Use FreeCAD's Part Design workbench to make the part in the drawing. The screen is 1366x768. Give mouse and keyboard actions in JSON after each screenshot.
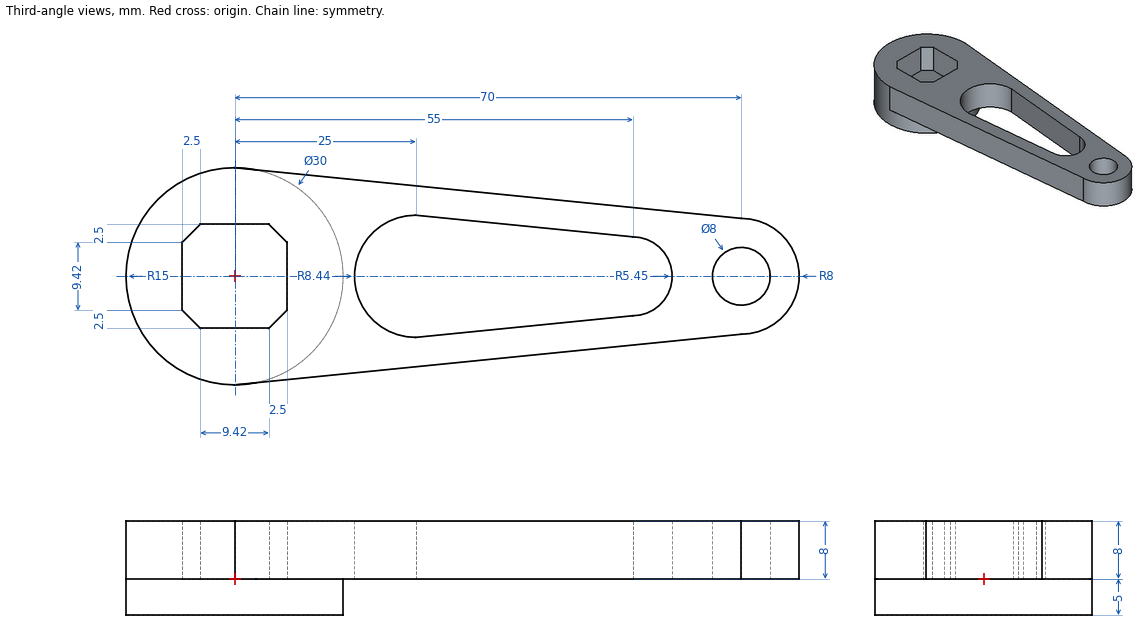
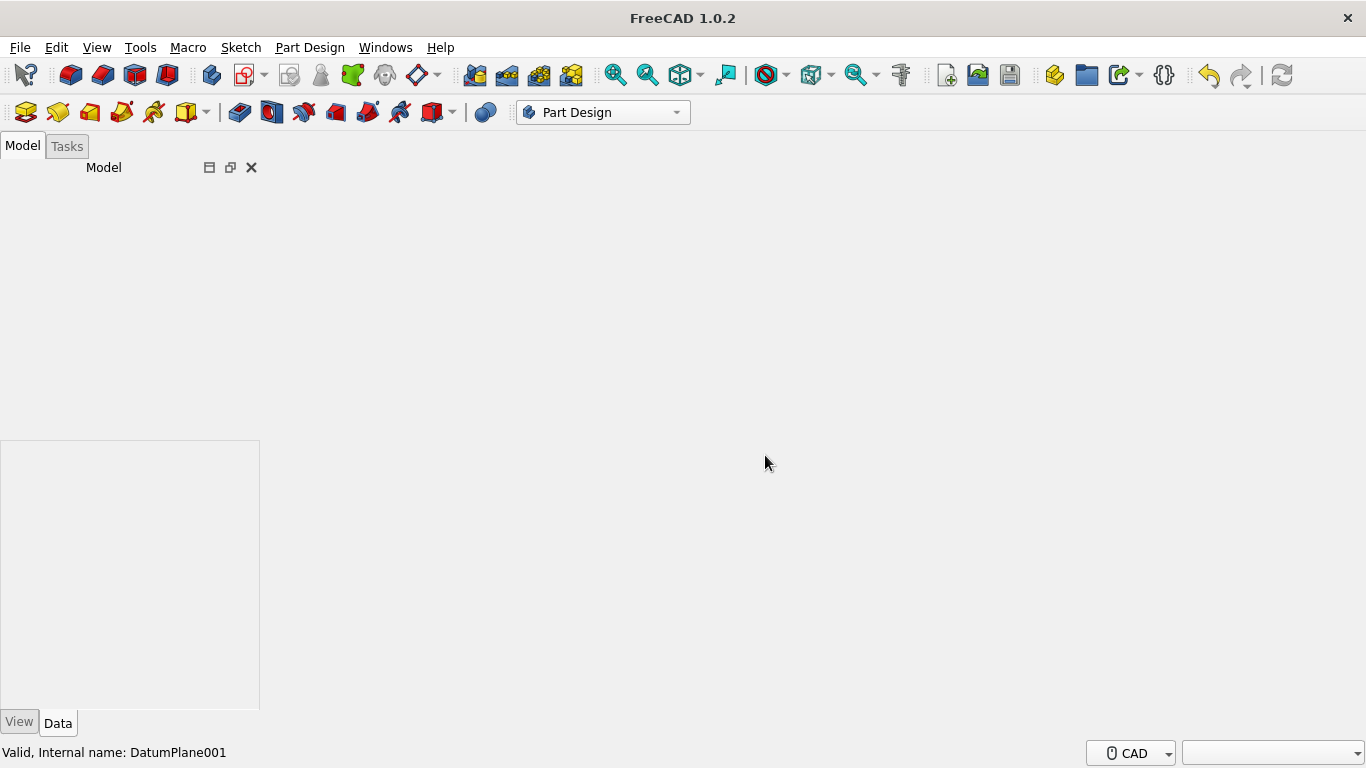
{"action": "left_click", "coordinate": [946, 76]}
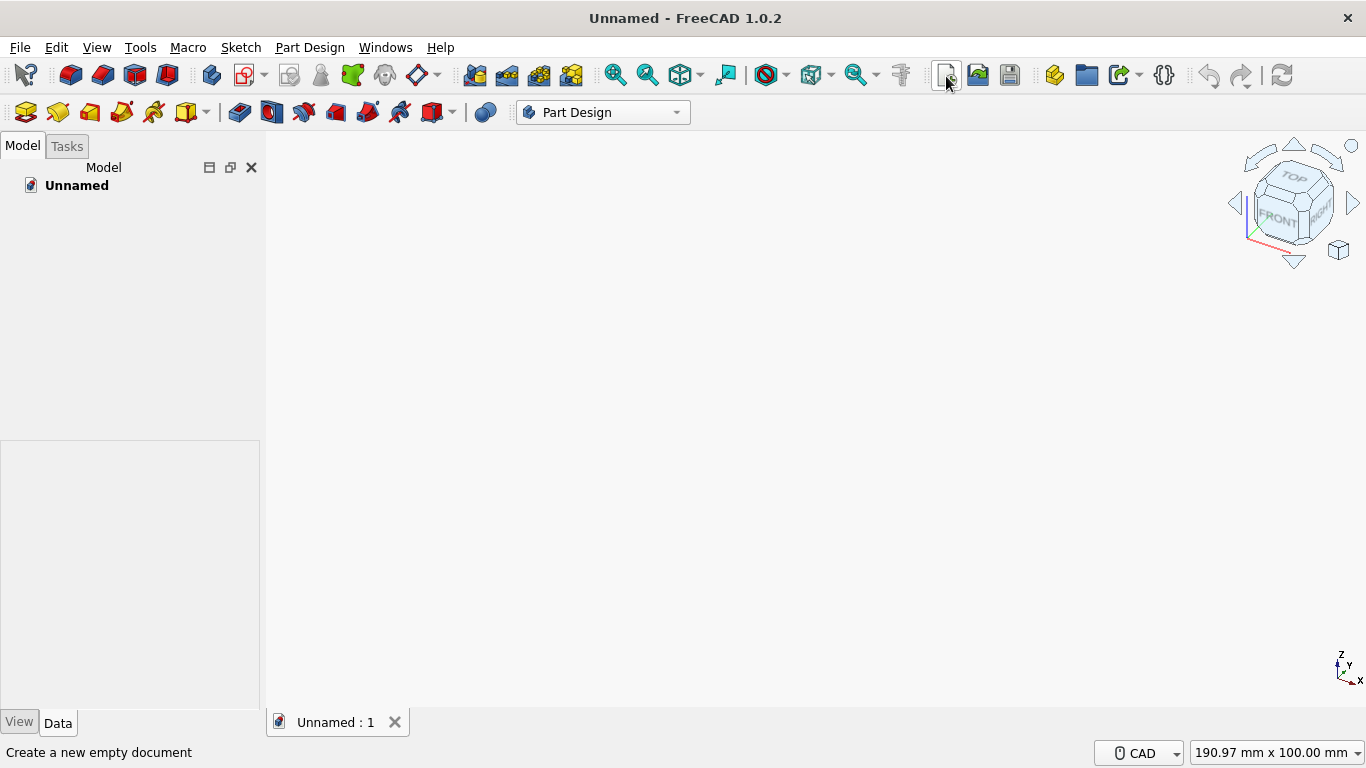
{"action": "left_click", "coordinate": [244, 76]}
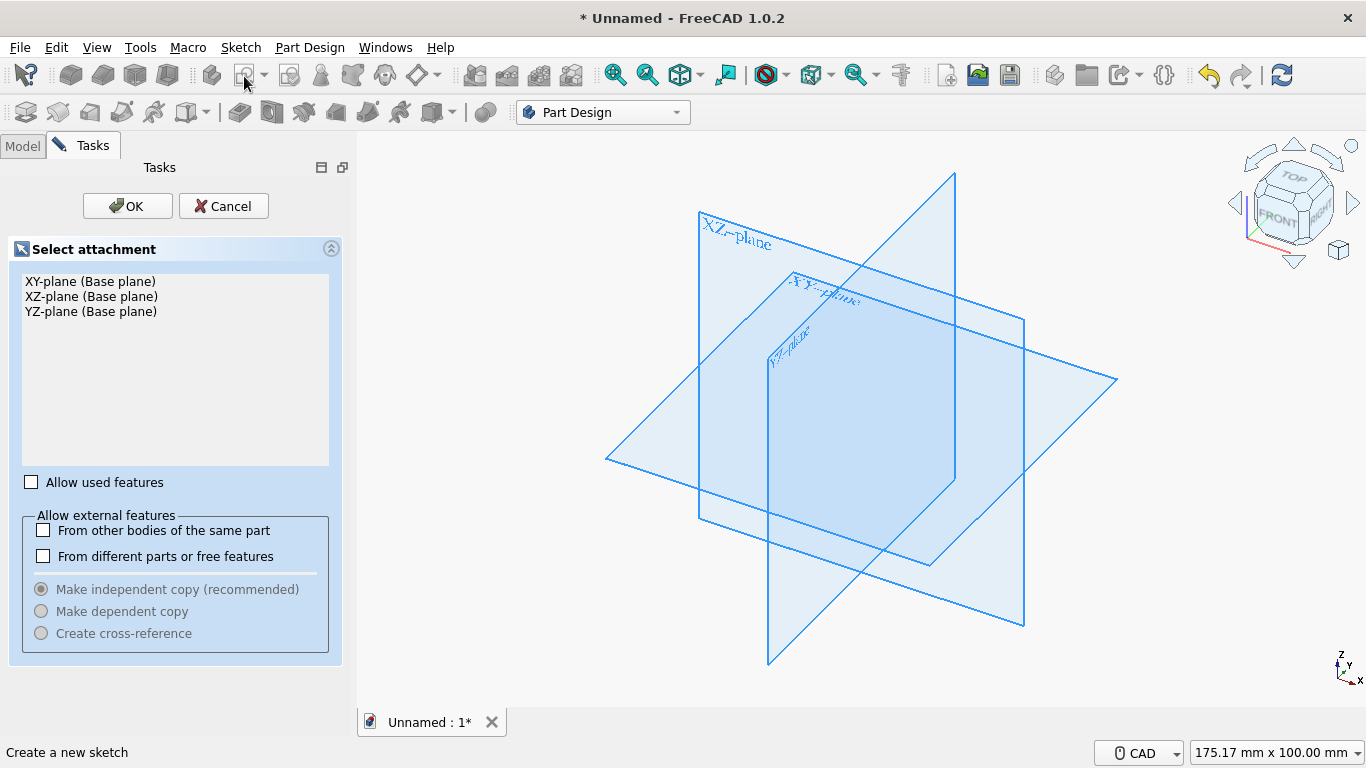
{"action": "left_click", "coordinate": [82, 282]}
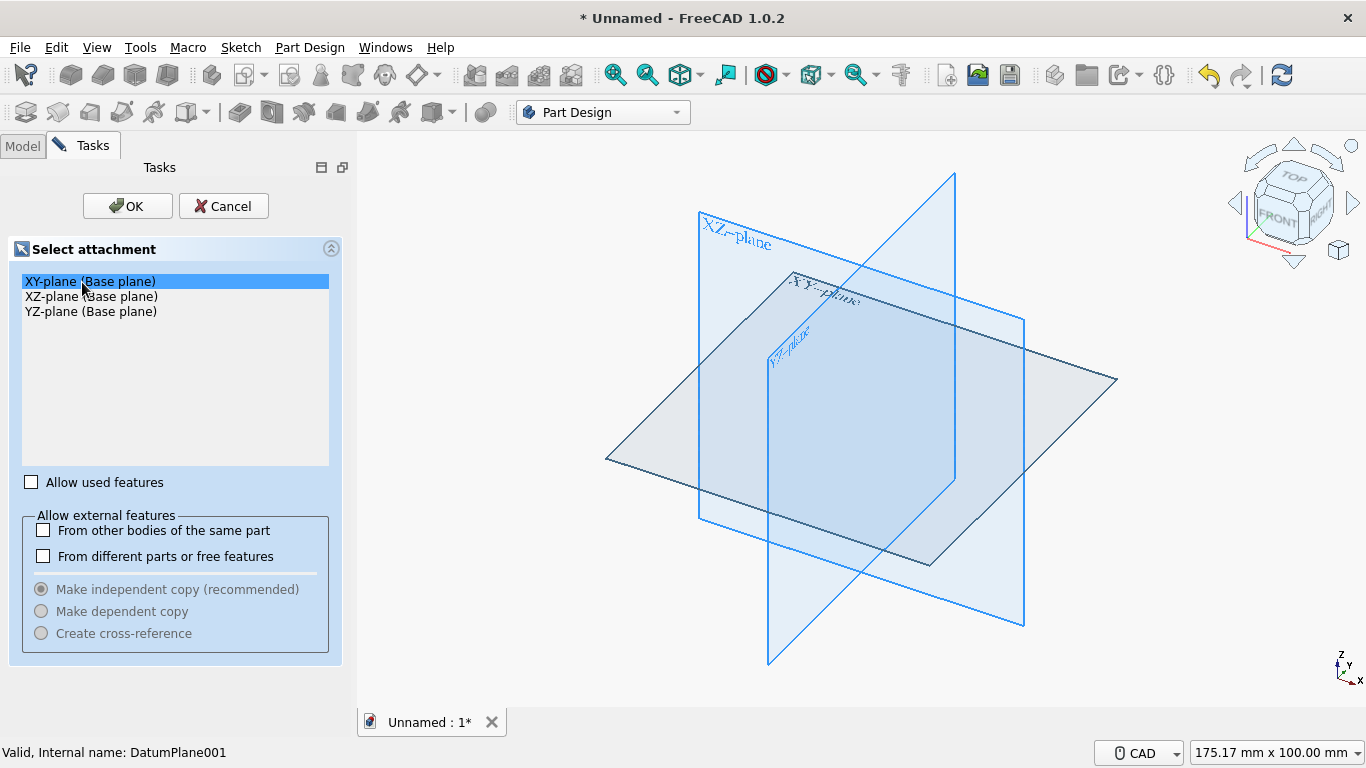
{"action": "left_click", "coordinate": [128, 206]}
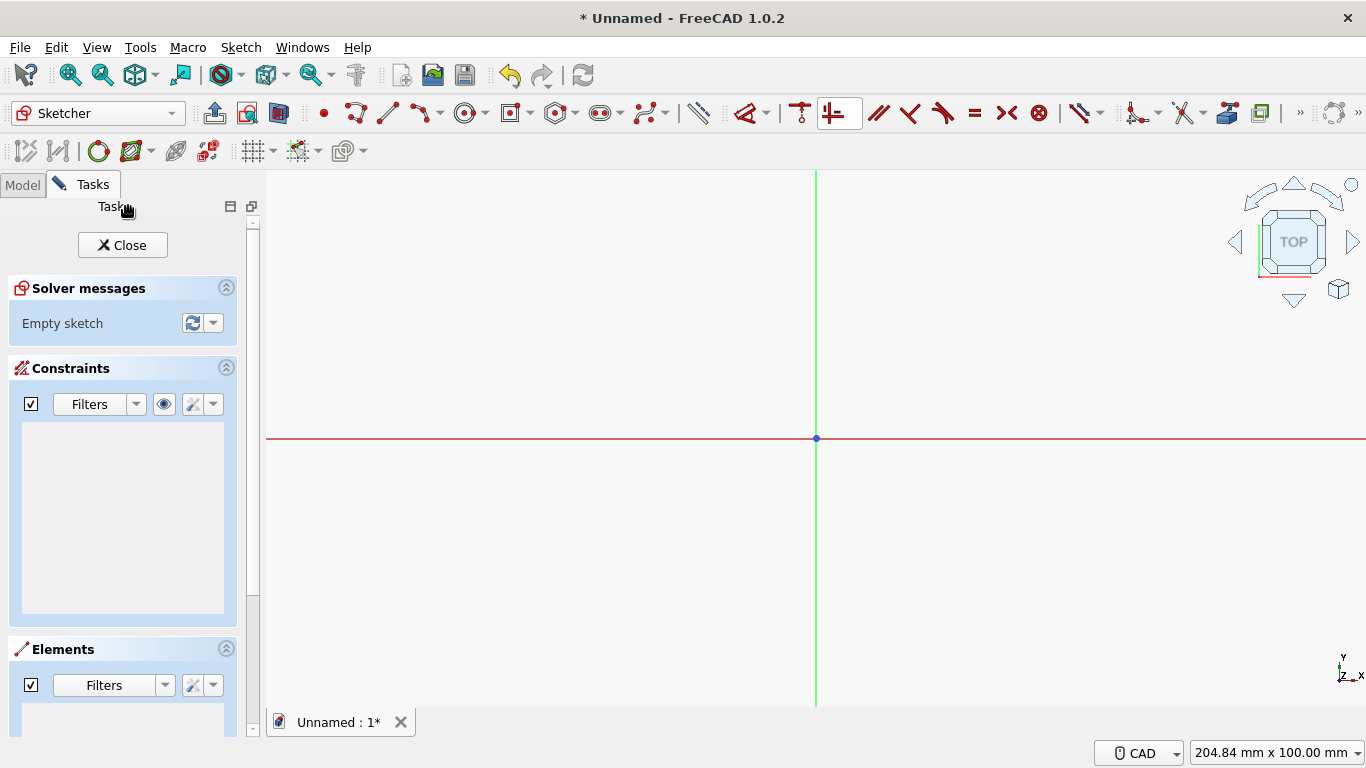
{"action": "scroll", "coordinate": [294, 439], "scroll_direction": "down", "scroll_amount": 1}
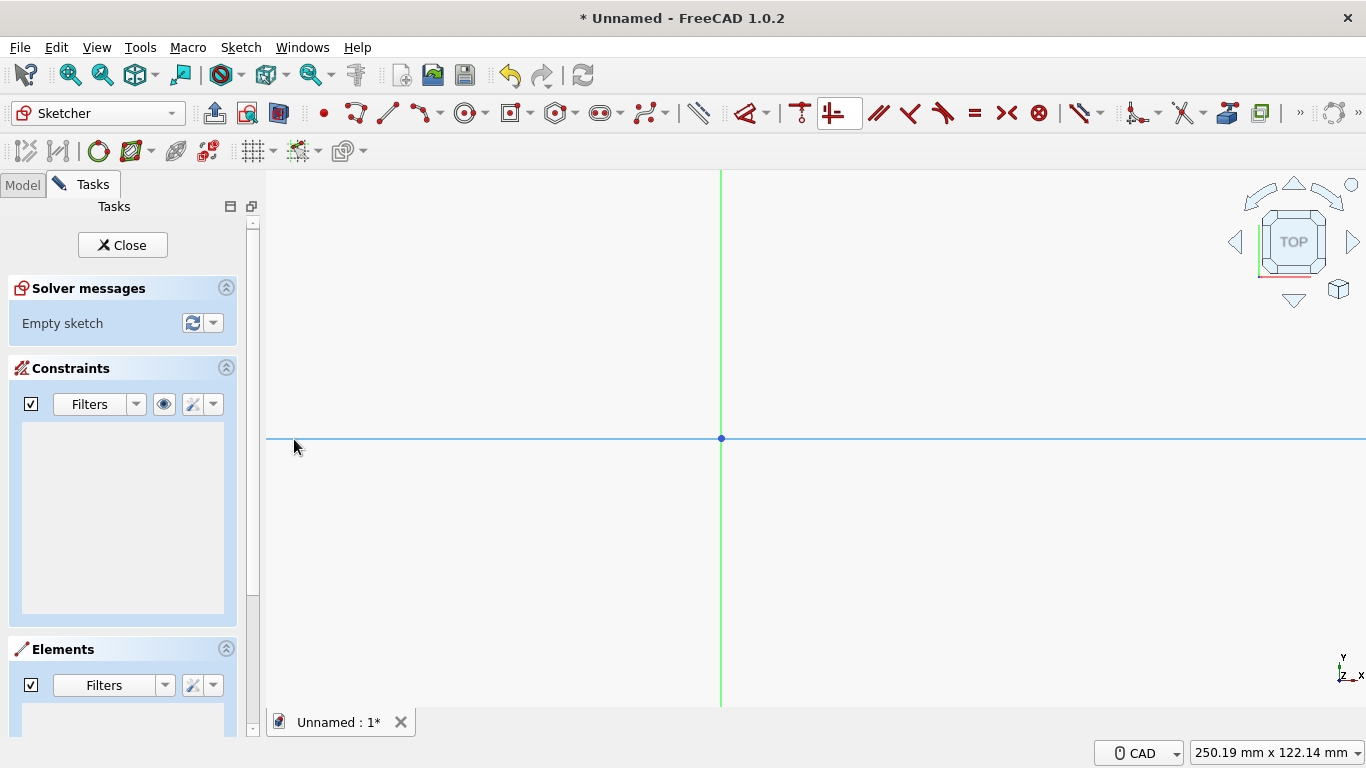
{"action": "scroll", "coordinate": [1088, 439], "scroll_direction": "up", "scroll_amount": 2}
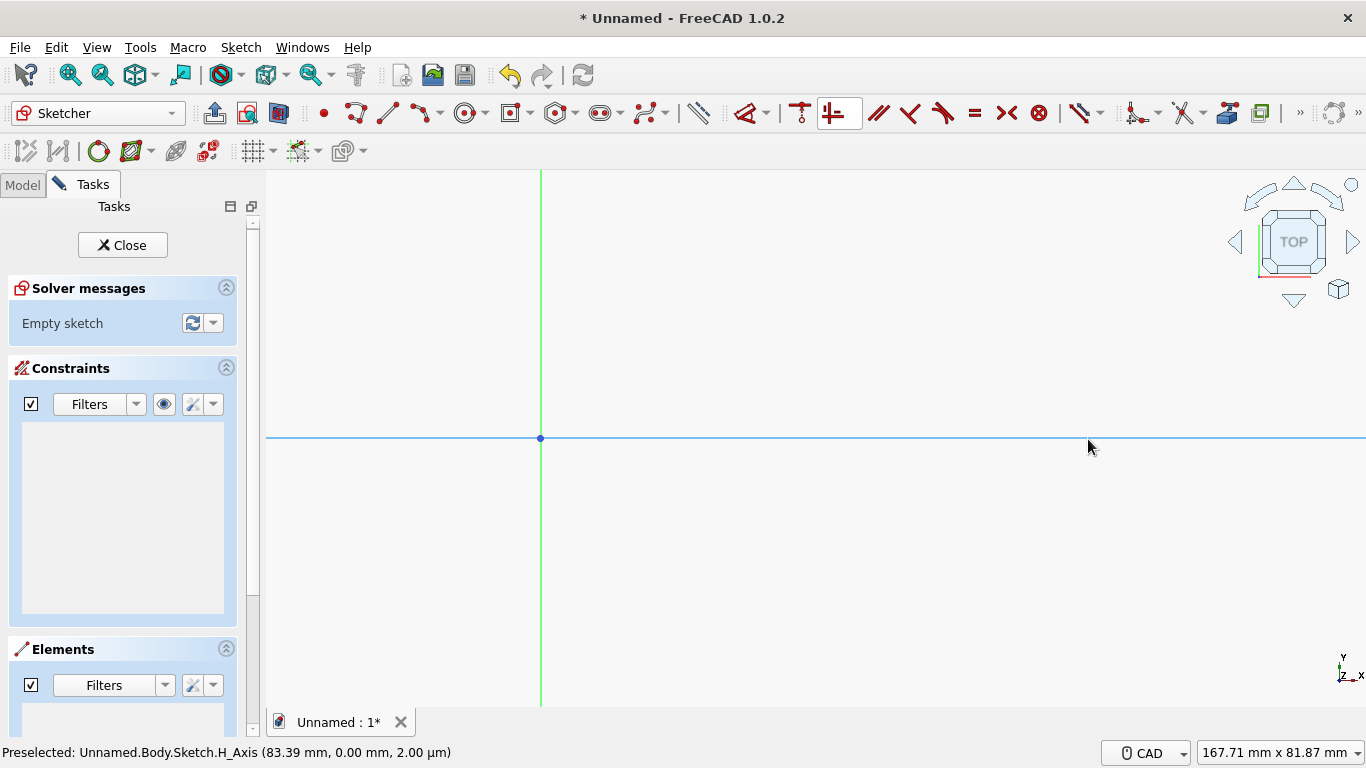
{"action": "left_click", "coordinate": [388, 114]}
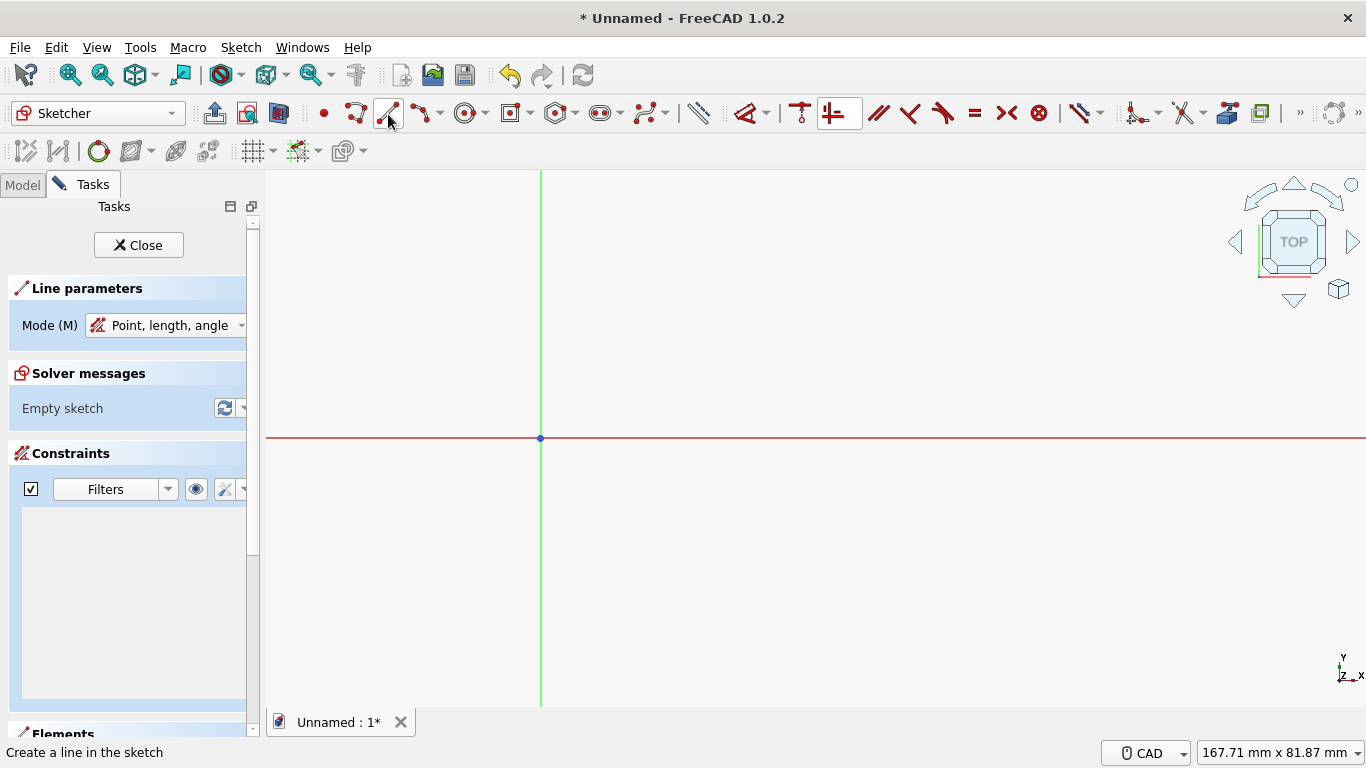
{"action": "left_click", "coordinate": [1000, 386]}
{"action": "left_click", "coordinate": [541, 340]}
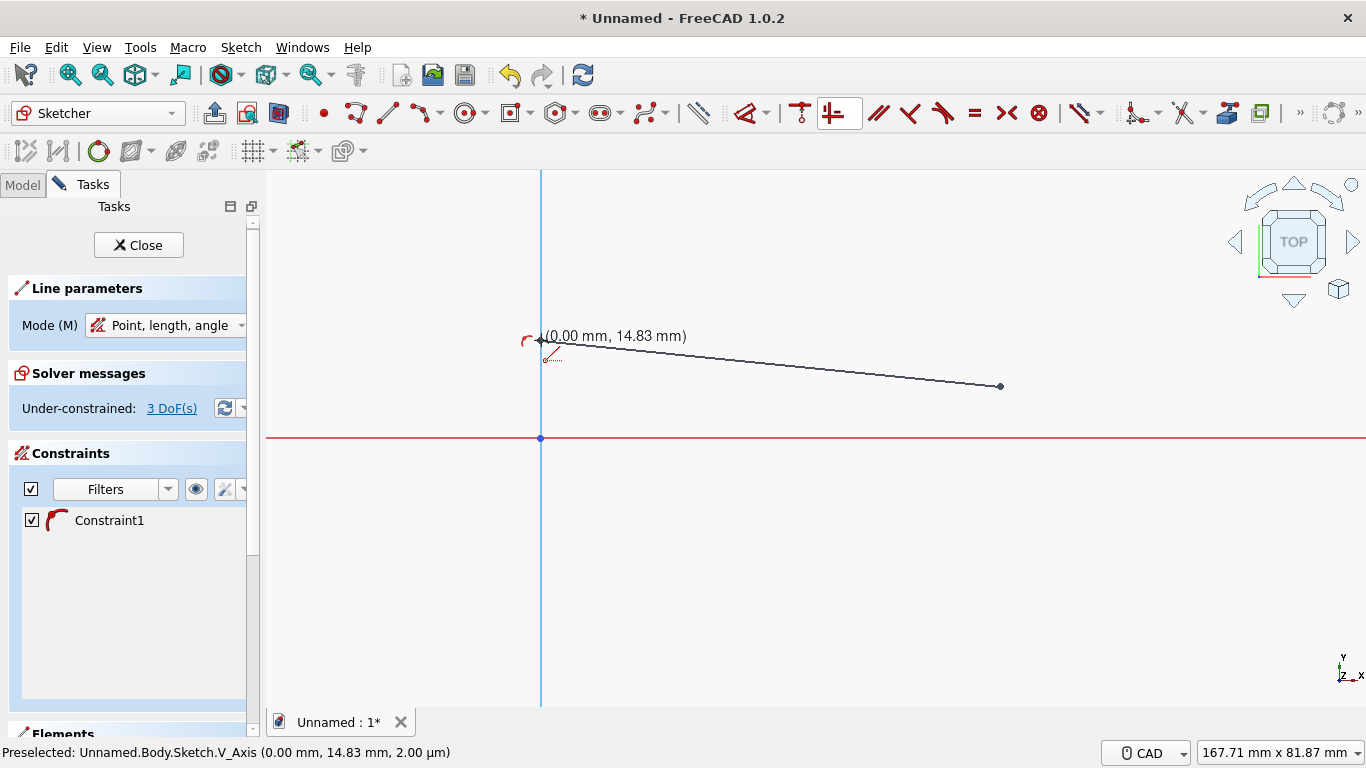
{"action": "left_click", "coordinate": [541, 537]}
{"action": "left_click", "coordinate": [1000, 491]}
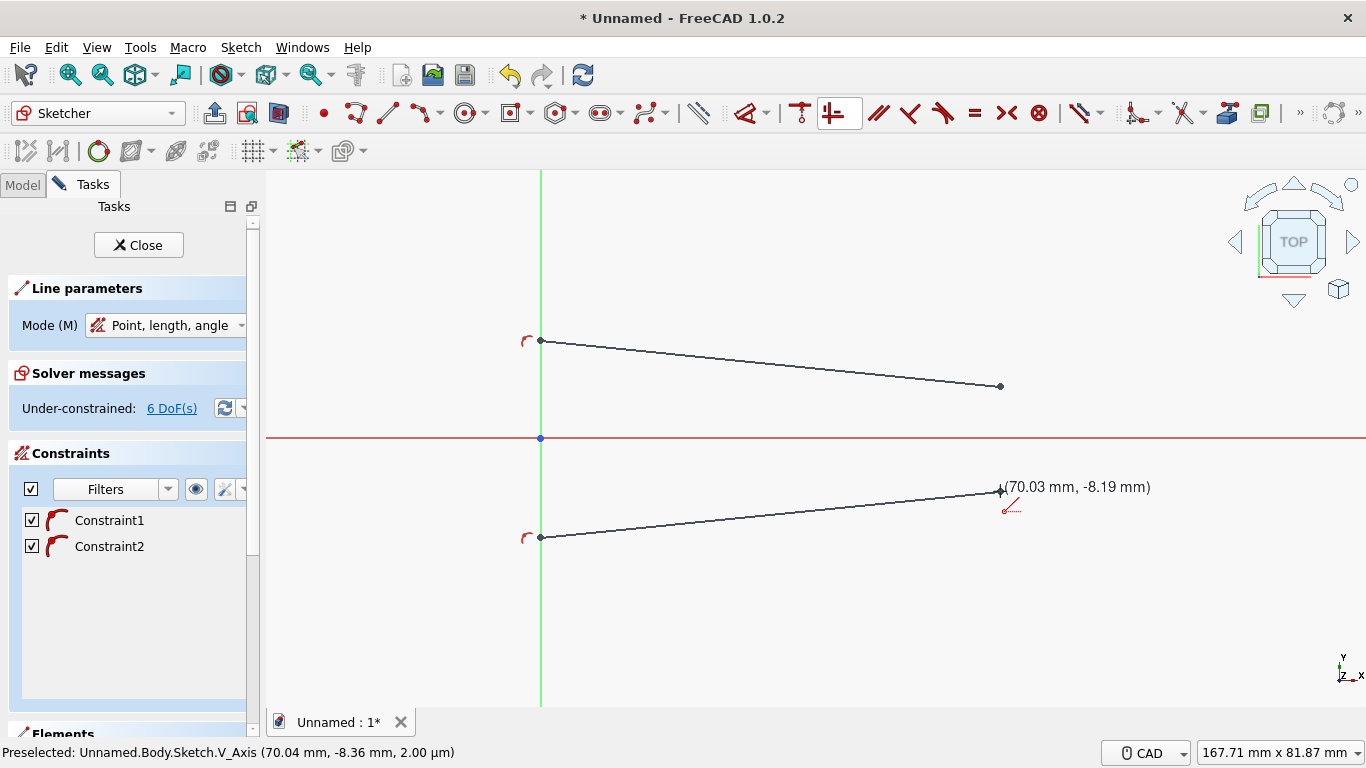
{"action": "left_click", "coordinate": [420, 114]}